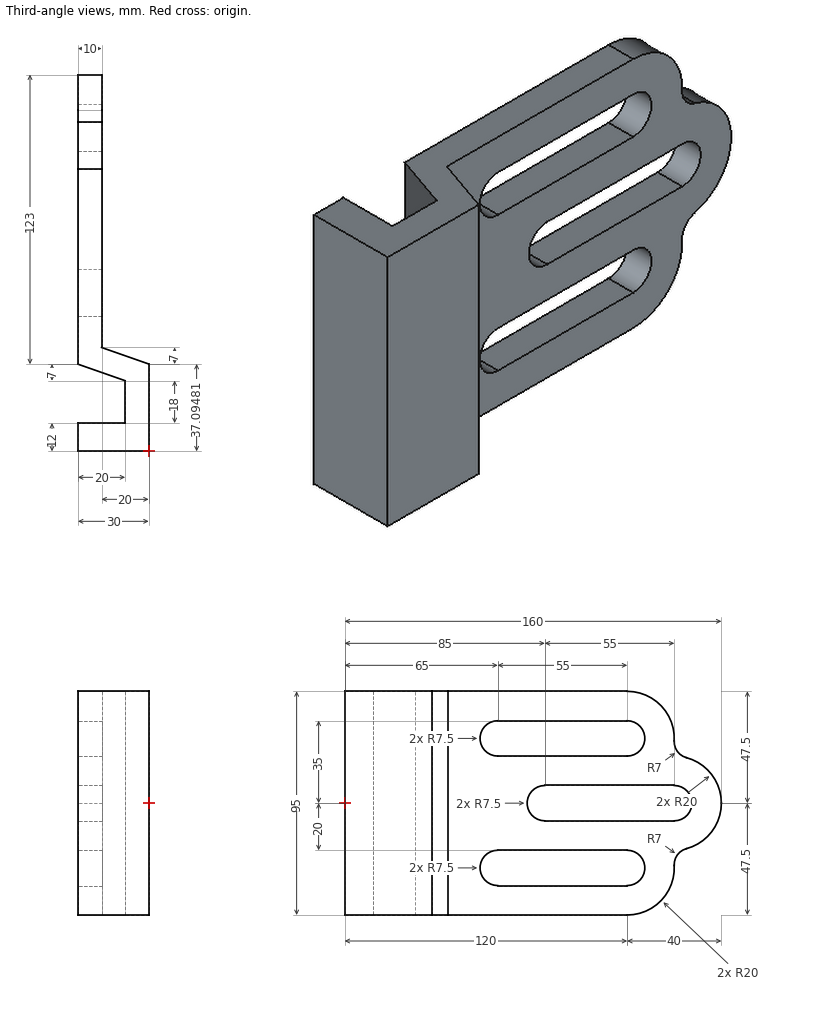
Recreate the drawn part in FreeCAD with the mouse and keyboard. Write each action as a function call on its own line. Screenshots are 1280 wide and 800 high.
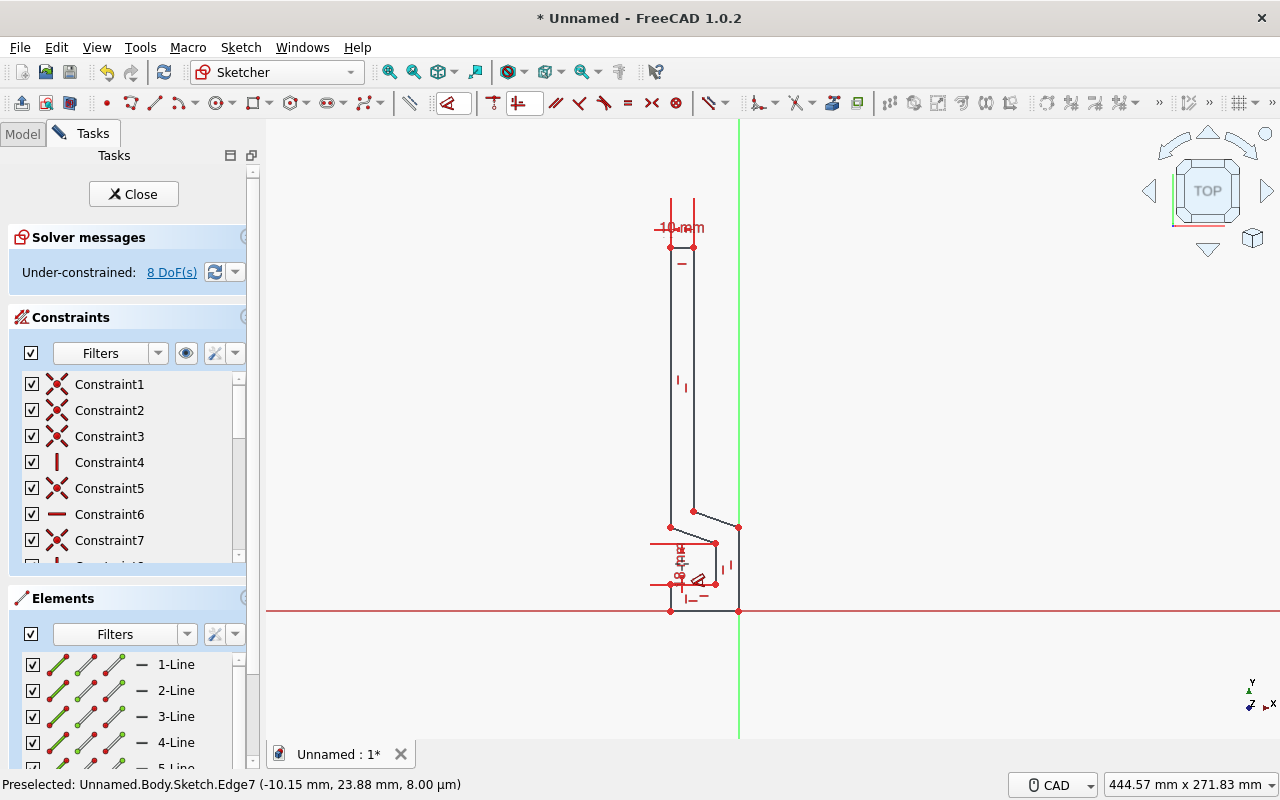
click(702, 585)
click(693, 643)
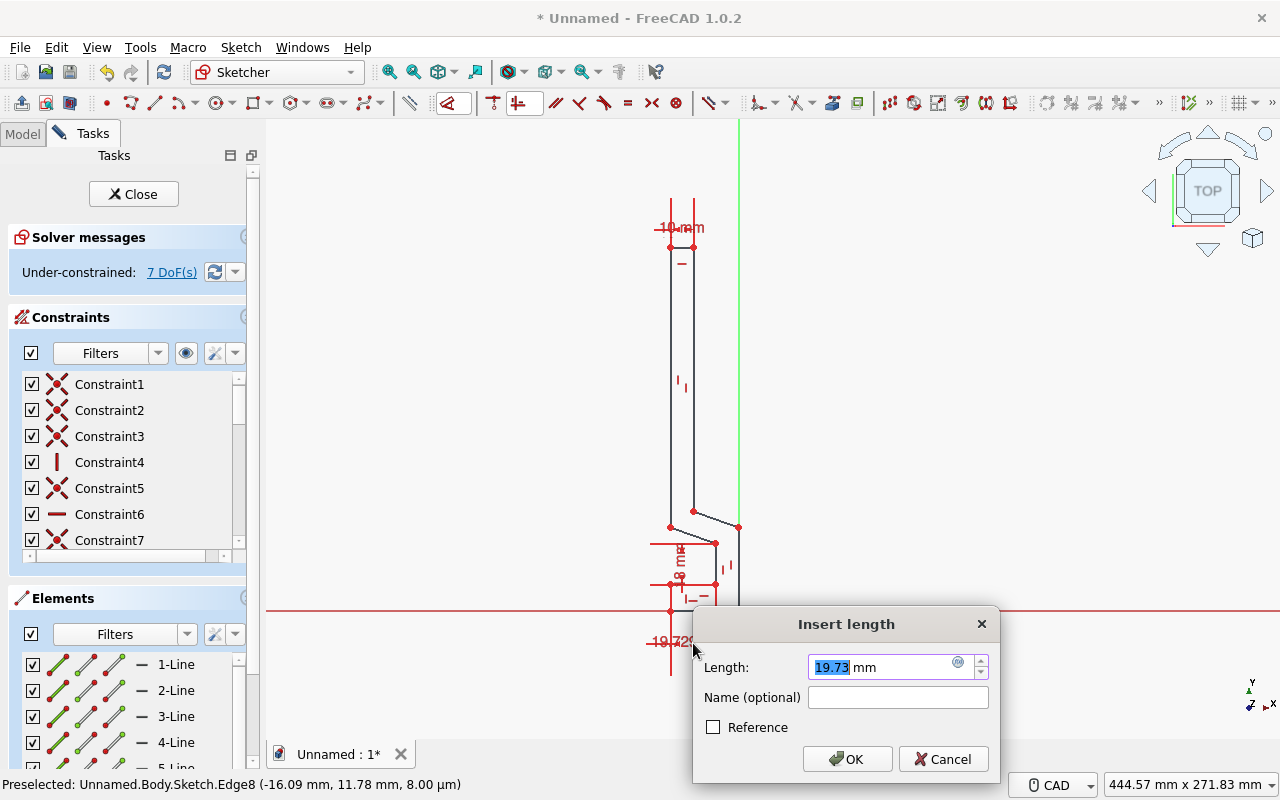
text(20)
key(Return)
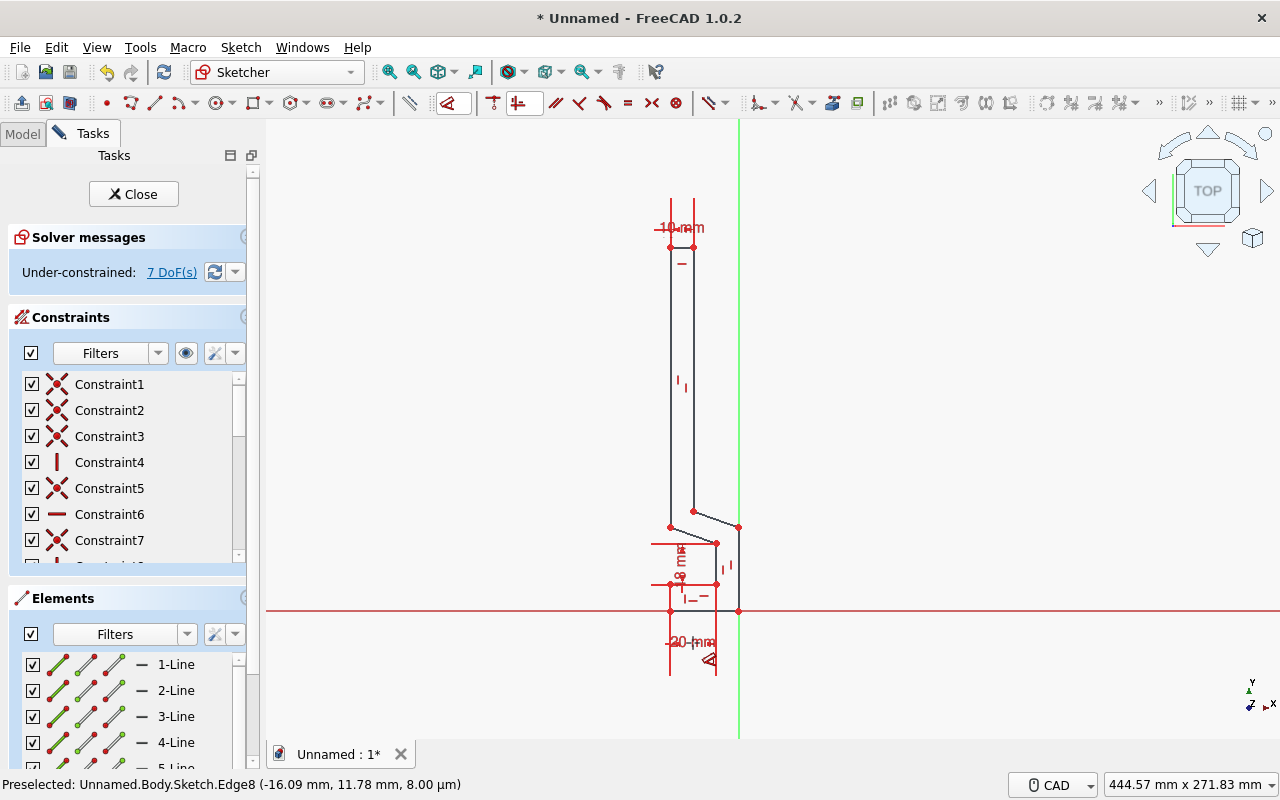
scroll(670, 595, up, 2)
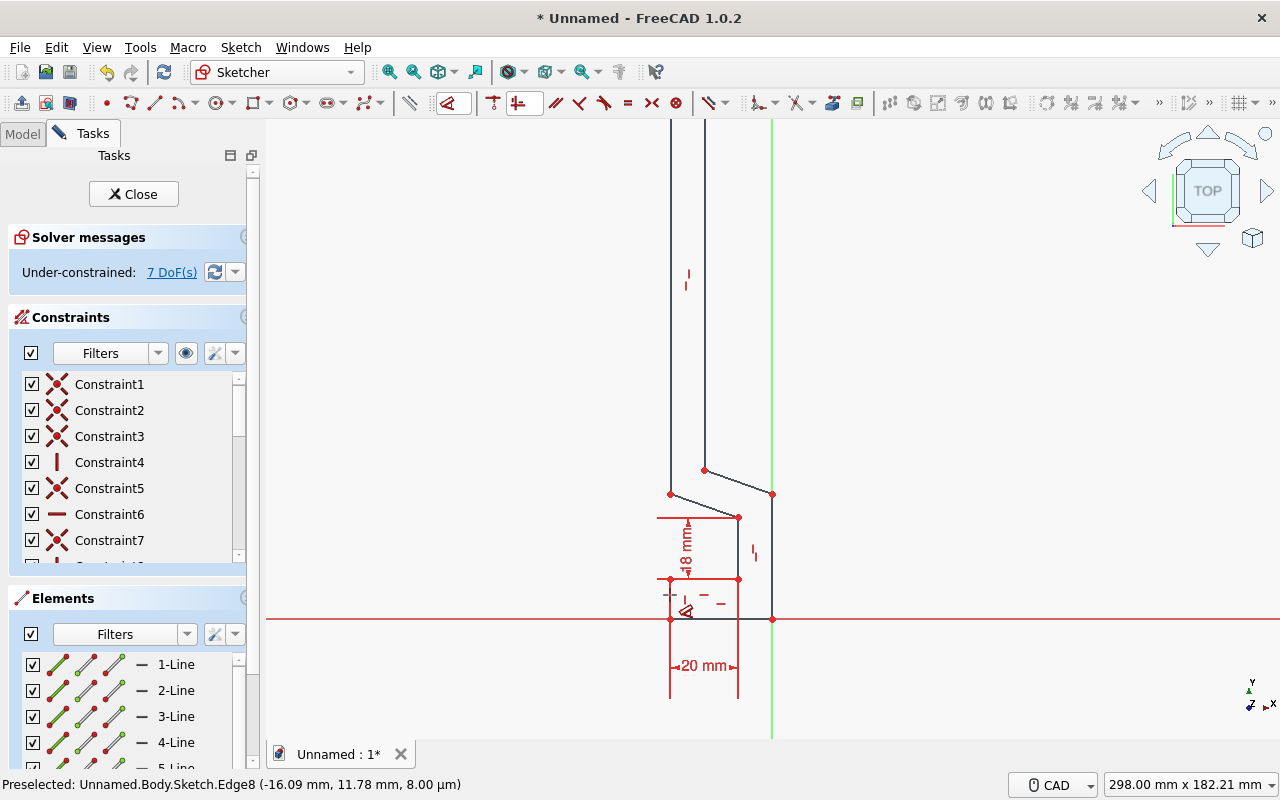
click(670, 595)
click(636, 599)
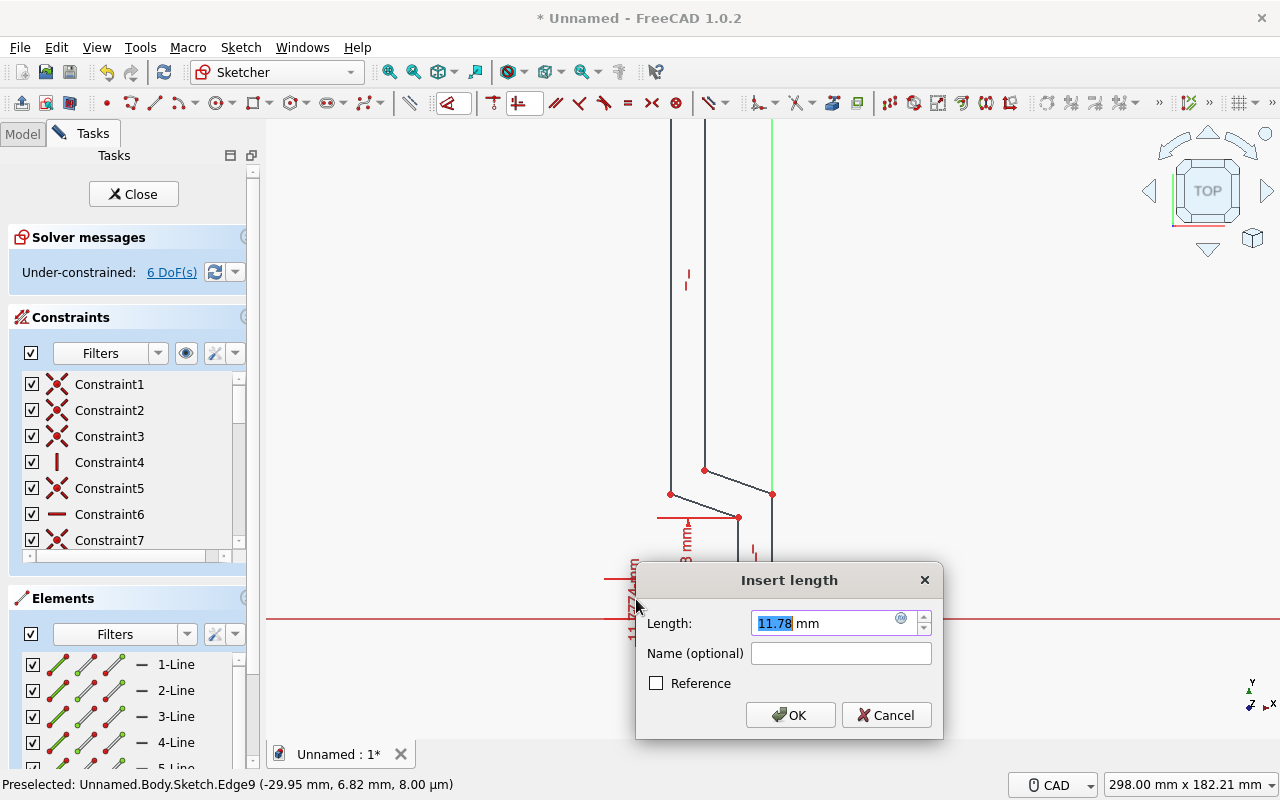
text(12)
key(Return)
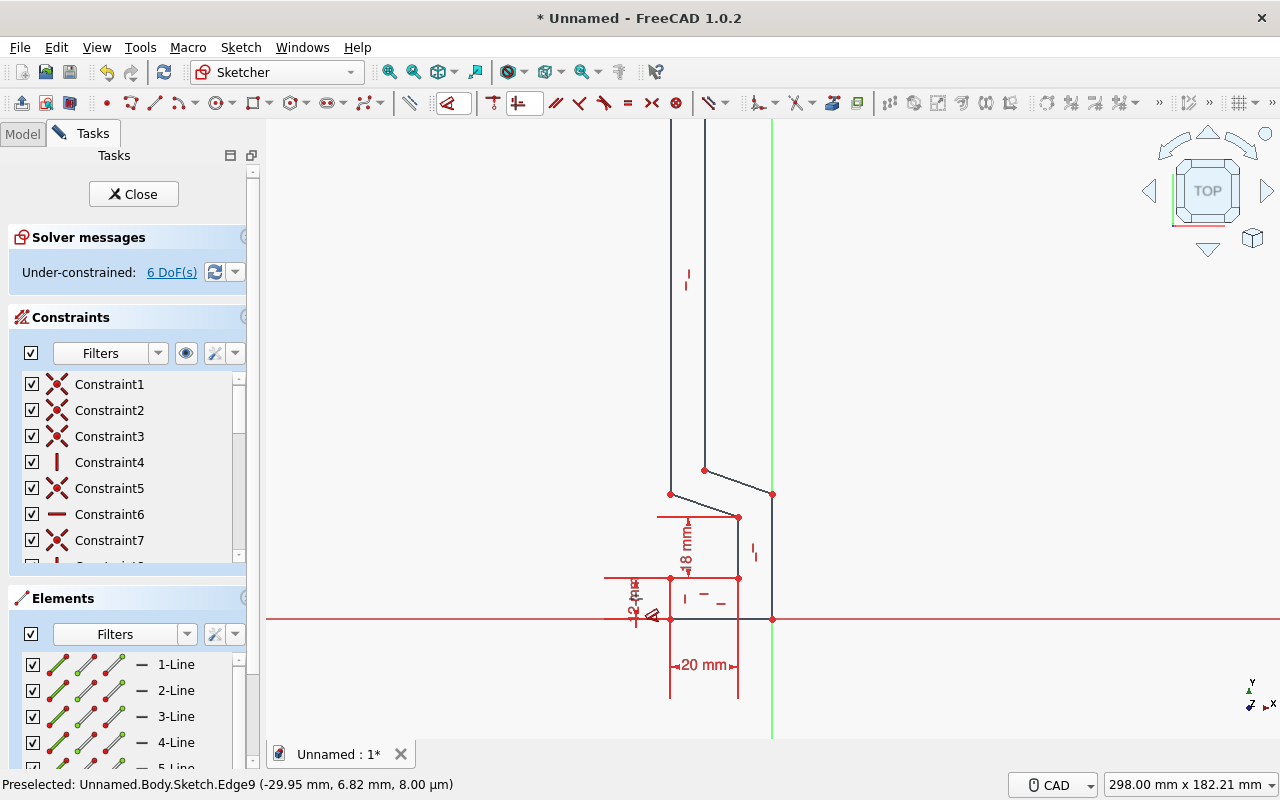
click(701, 619)
click(757, 585)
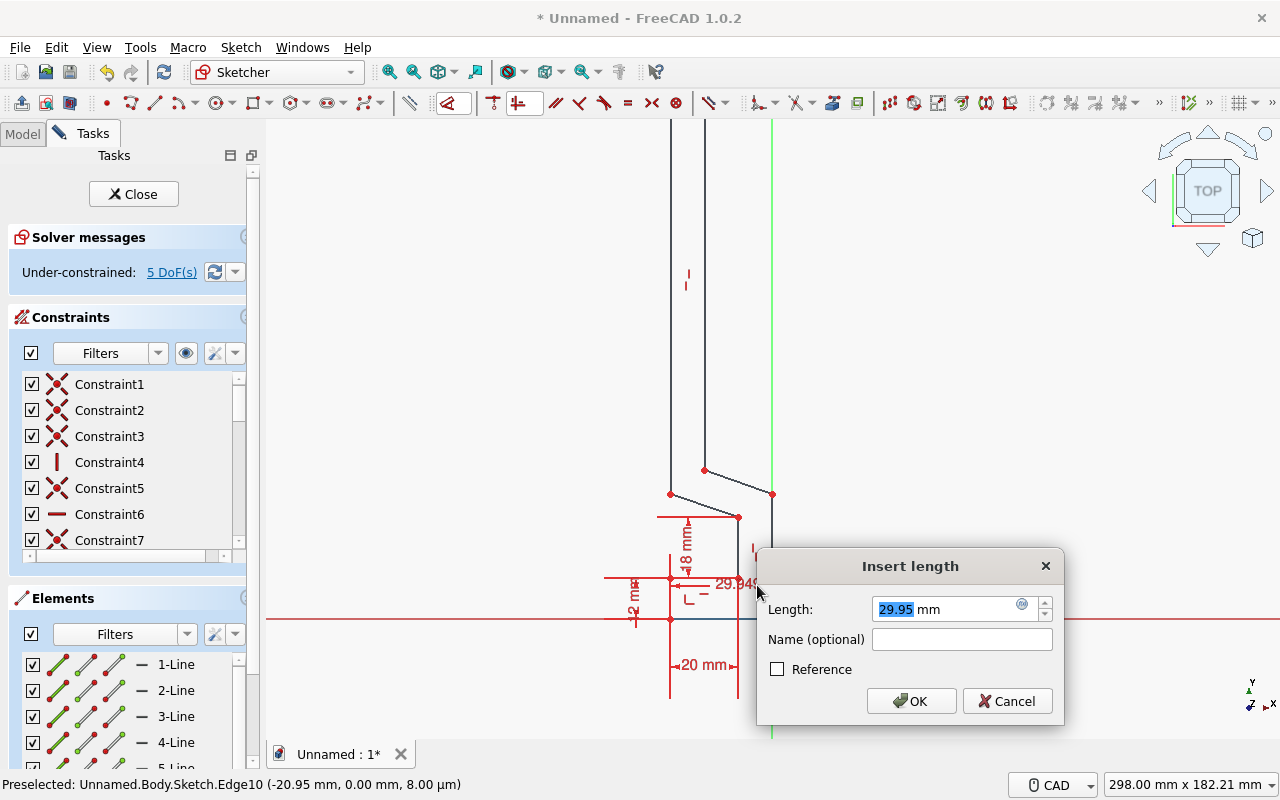
text(30)
key(Return)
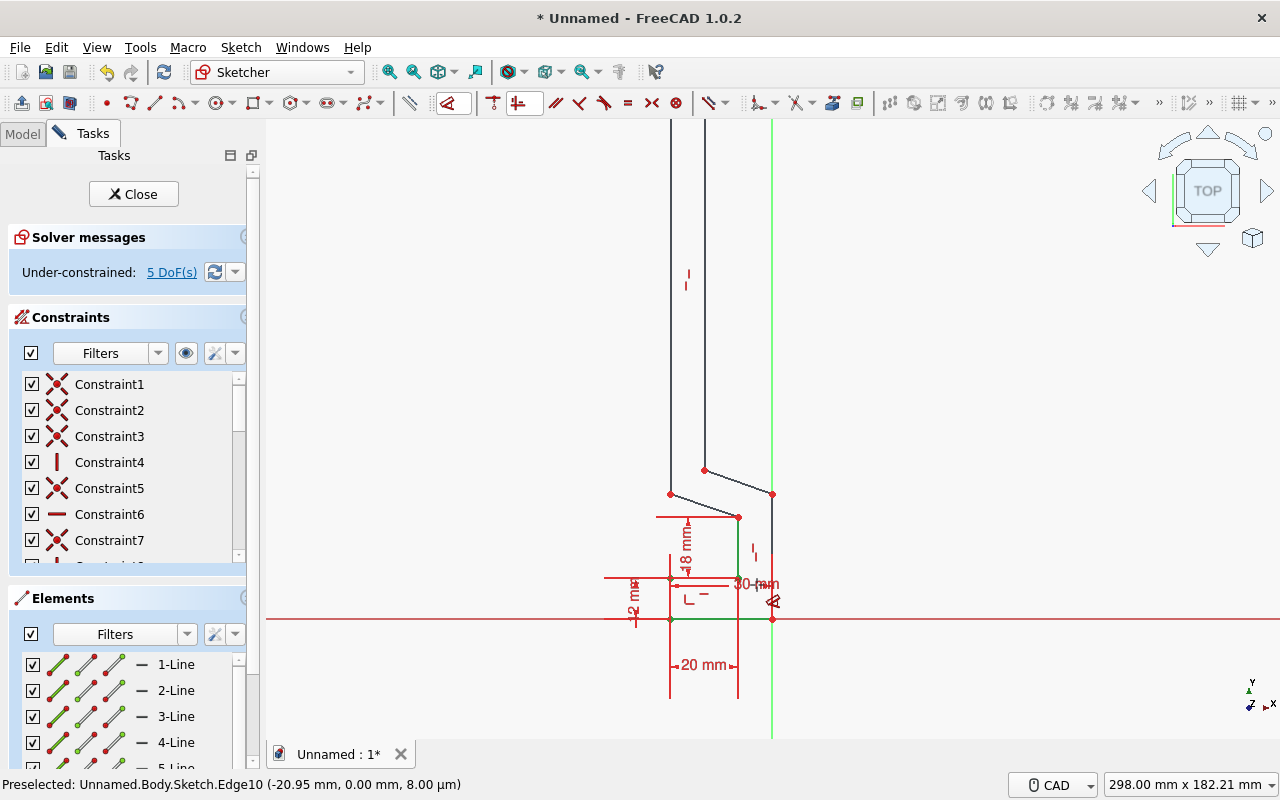
scroll(752, 487, up, 3)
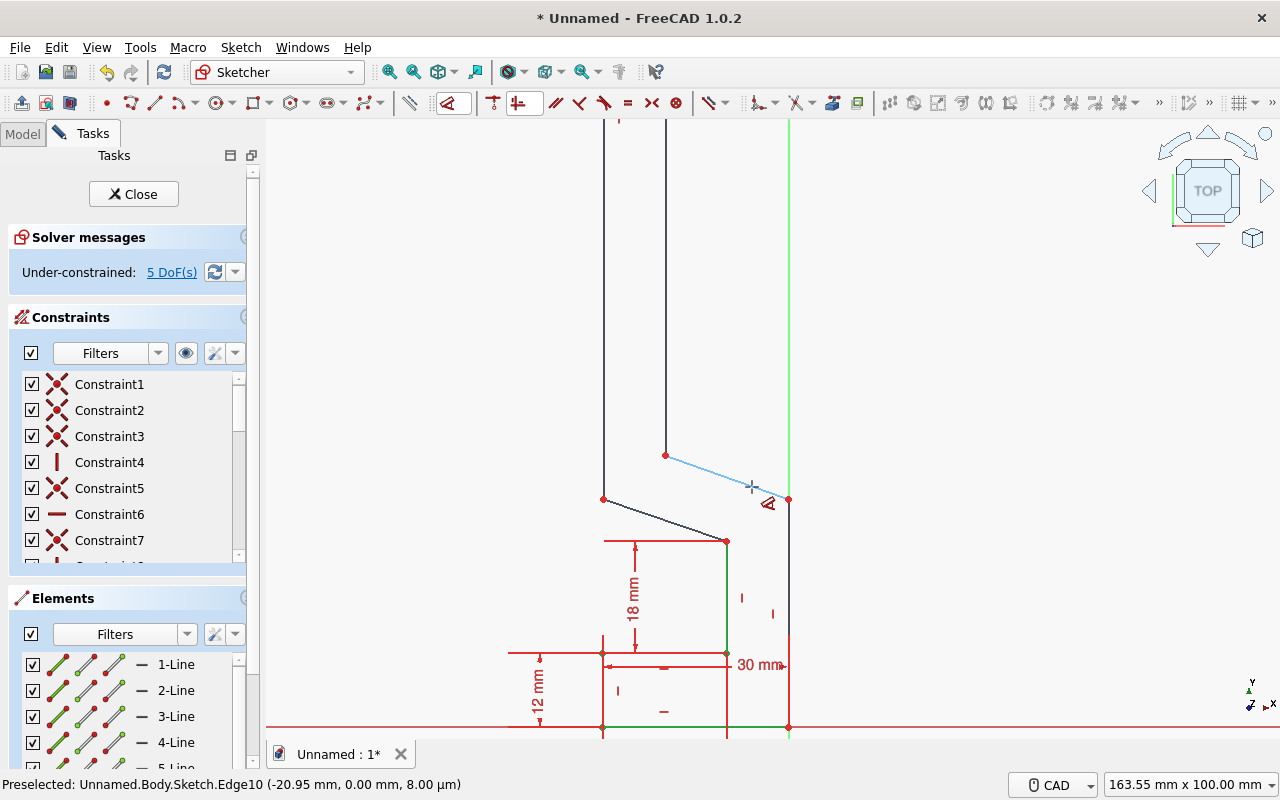
click(752, 486)
click(823, 478)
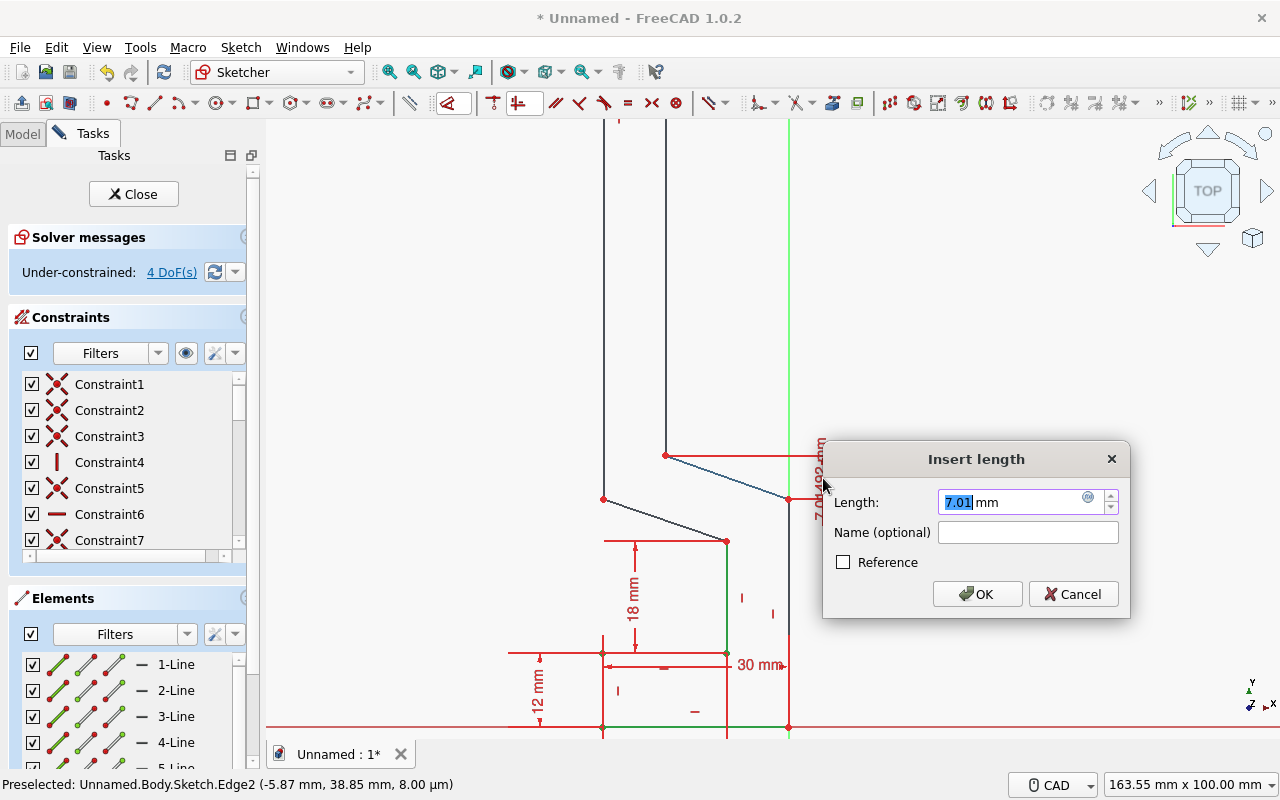
text(7)
key(Return)